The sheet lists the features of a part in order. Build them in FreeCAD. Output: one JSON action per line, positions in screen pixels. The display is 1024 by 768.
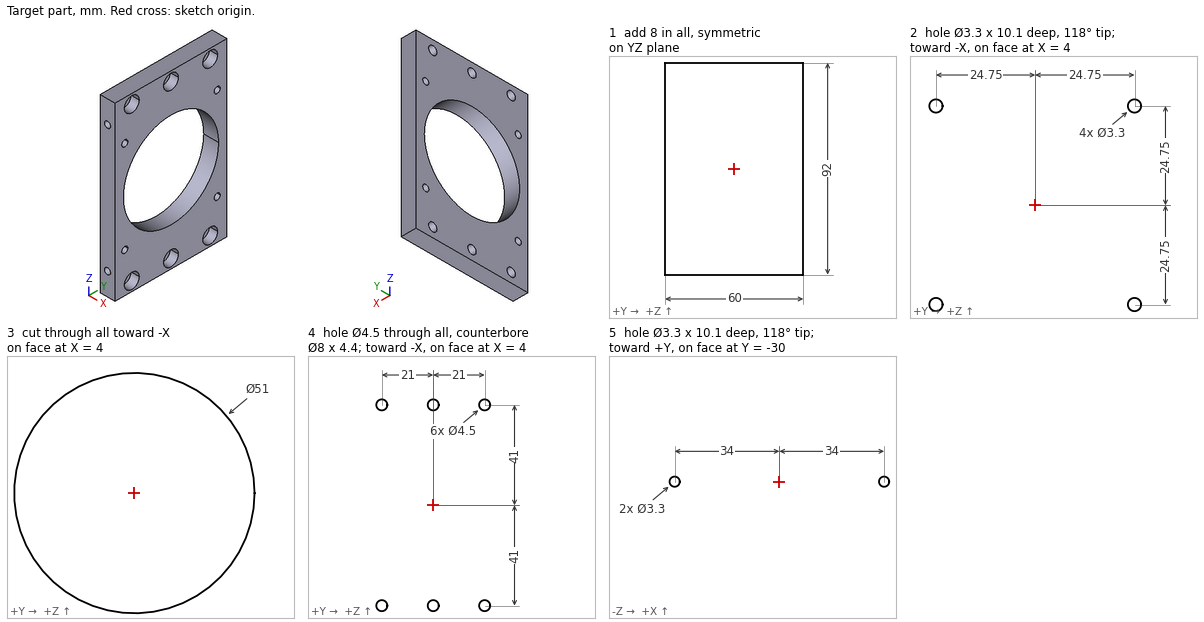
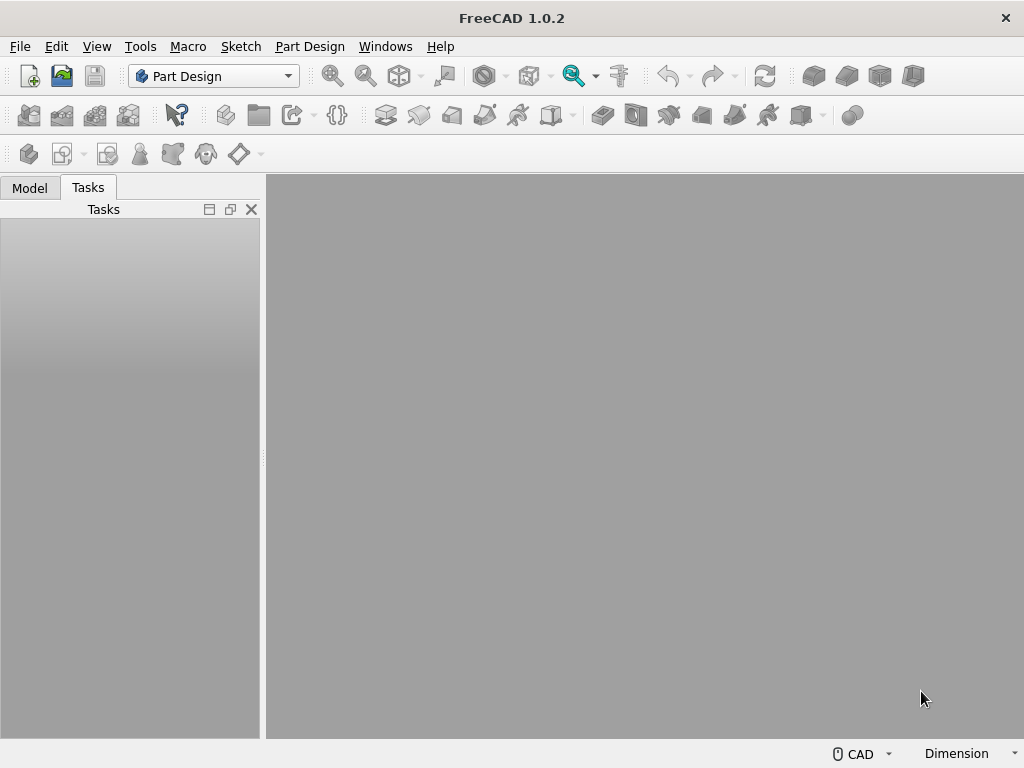
{"action": "left_click", "coordinate": [29, 76]}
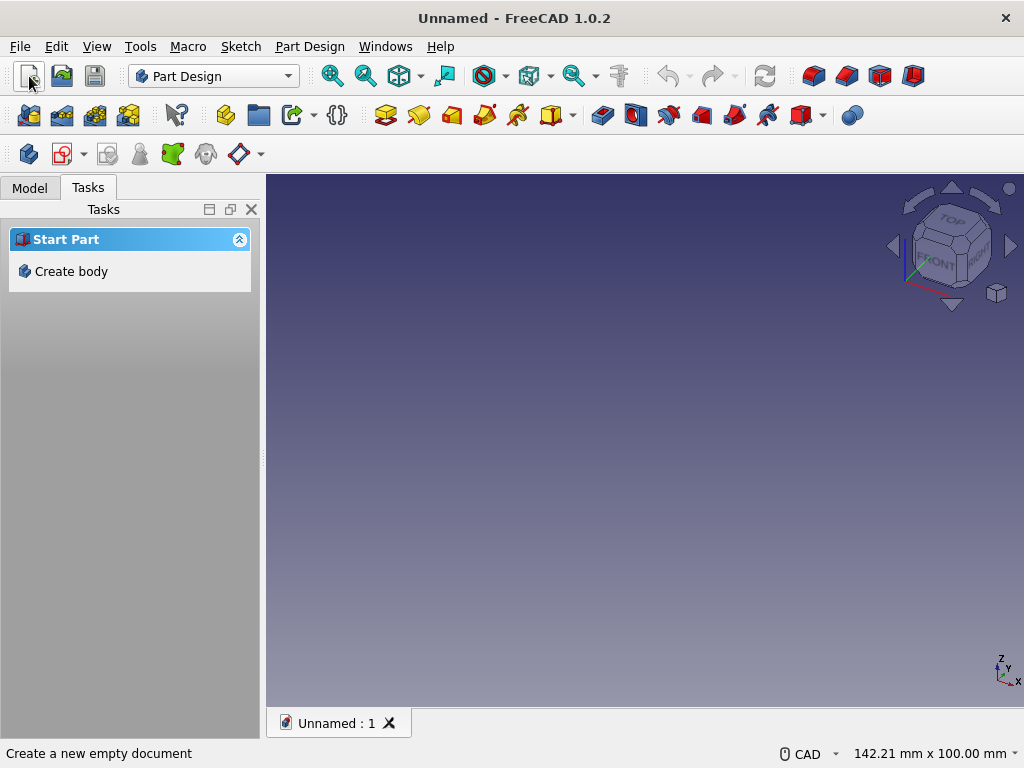
{"action": "left_click", "coordinate": [62, 154]}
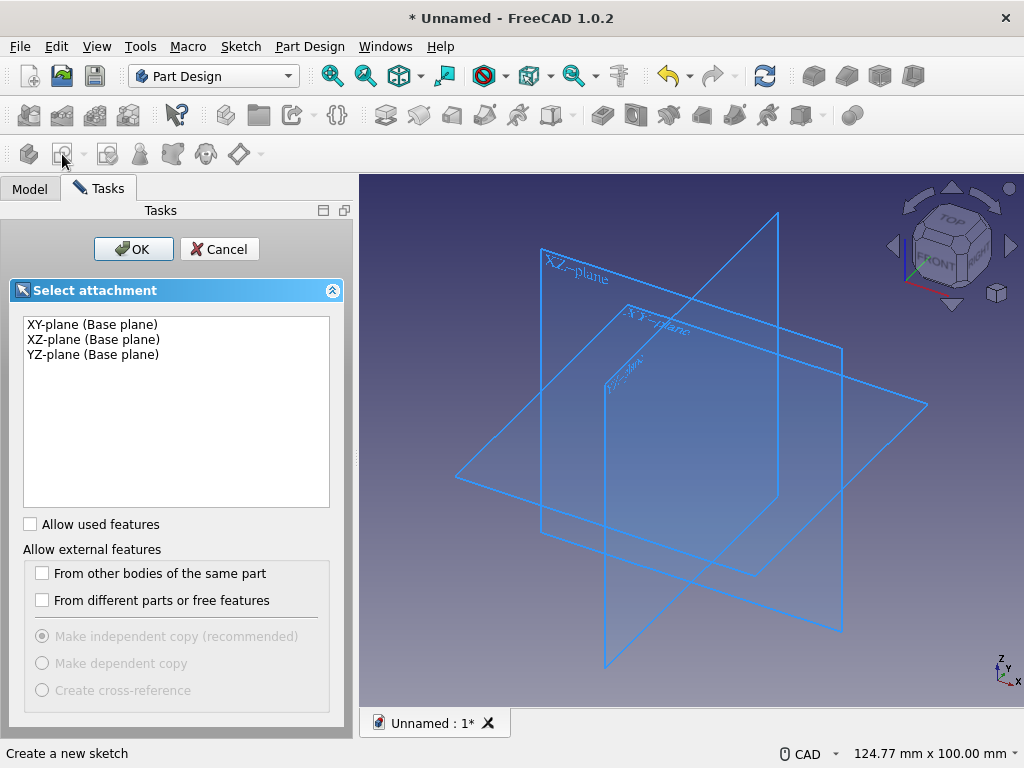
{"action": "left_click", "coordinate": [84, 354]}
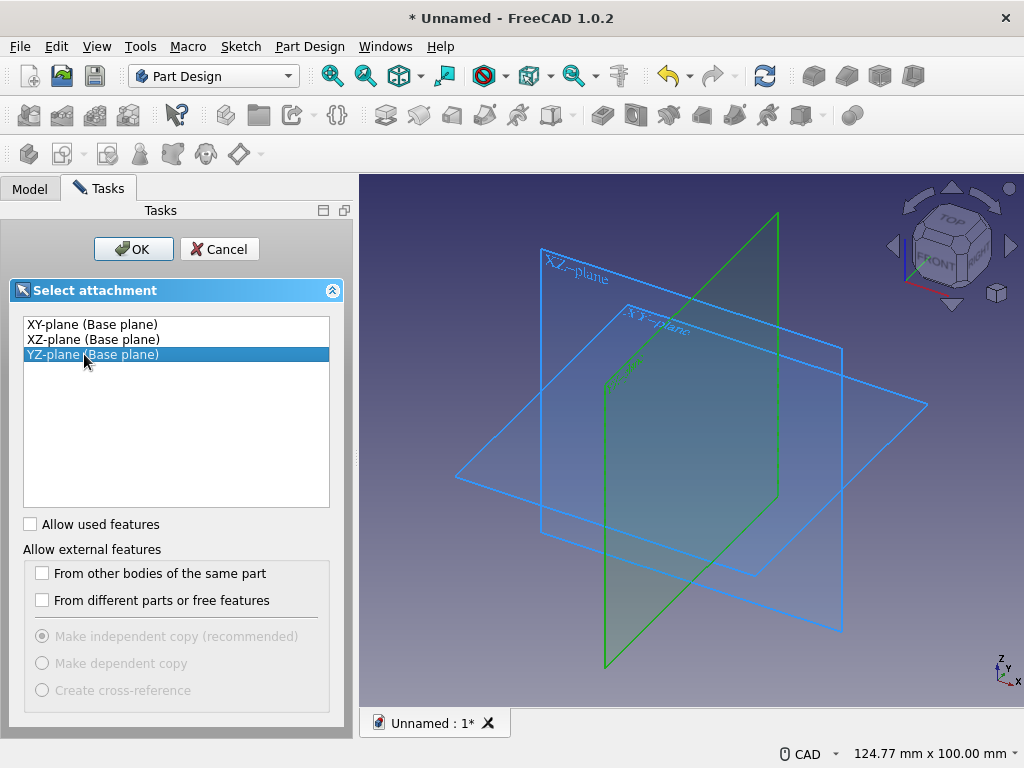
{"action": "left_click", "coordinate": [134, 249]}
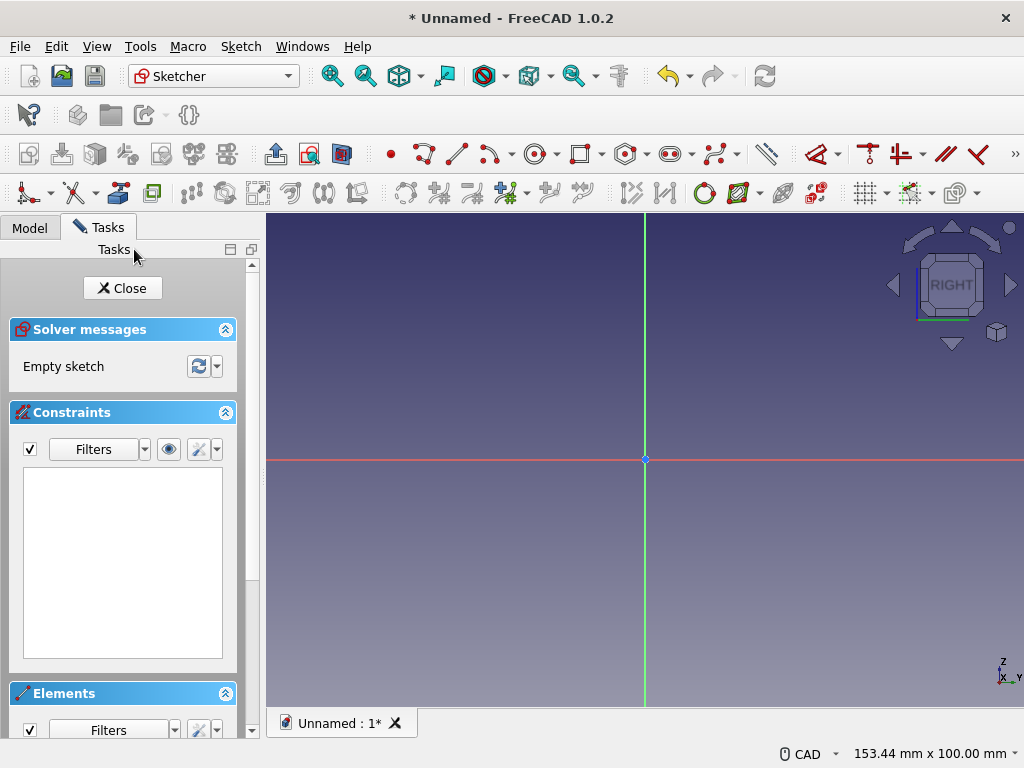
{"action": "scroll", "coordinate": [437, 460], "scroll_direction": "down", "scroll_amount": 2}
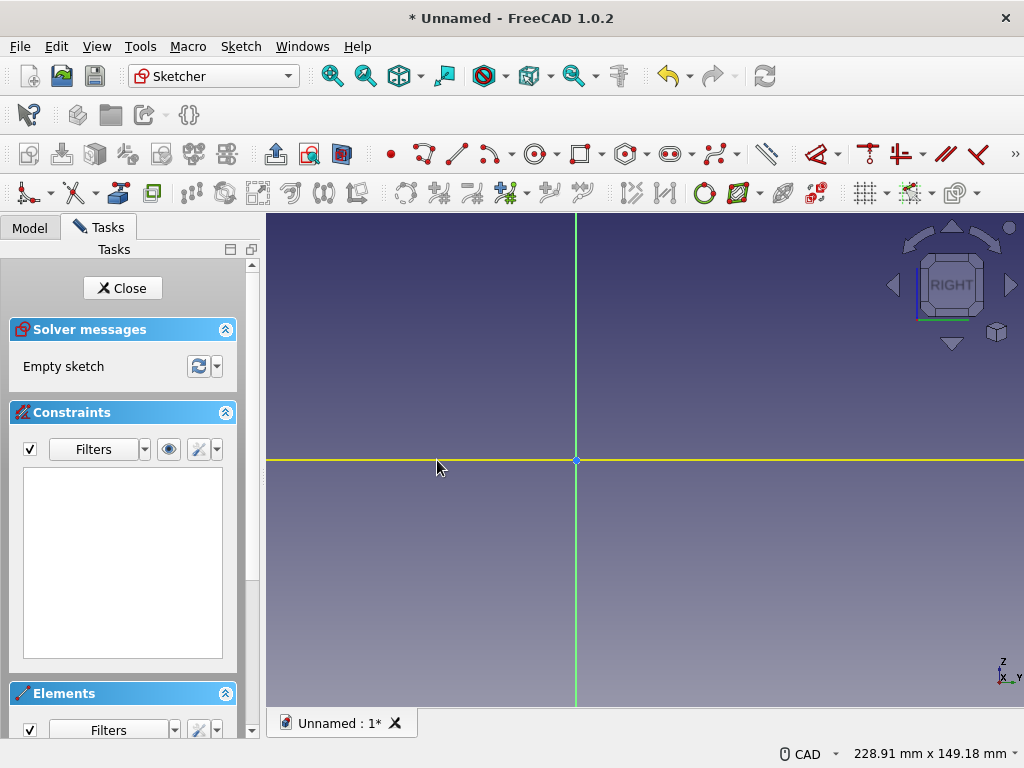
{"action": "key", "text": "g v"}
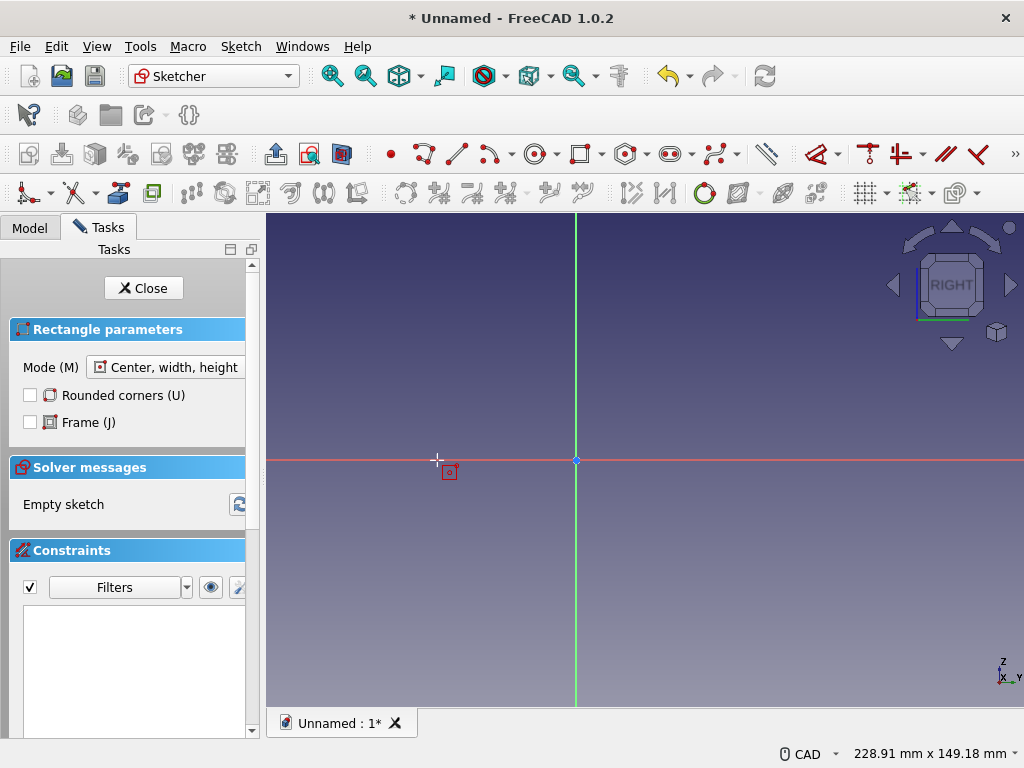
{"action": "left_click", "coordinate": [577, 460]}
{"action": "left_click", "coordinate": [676, 308]}
{"action": "key", "text": "Escape"}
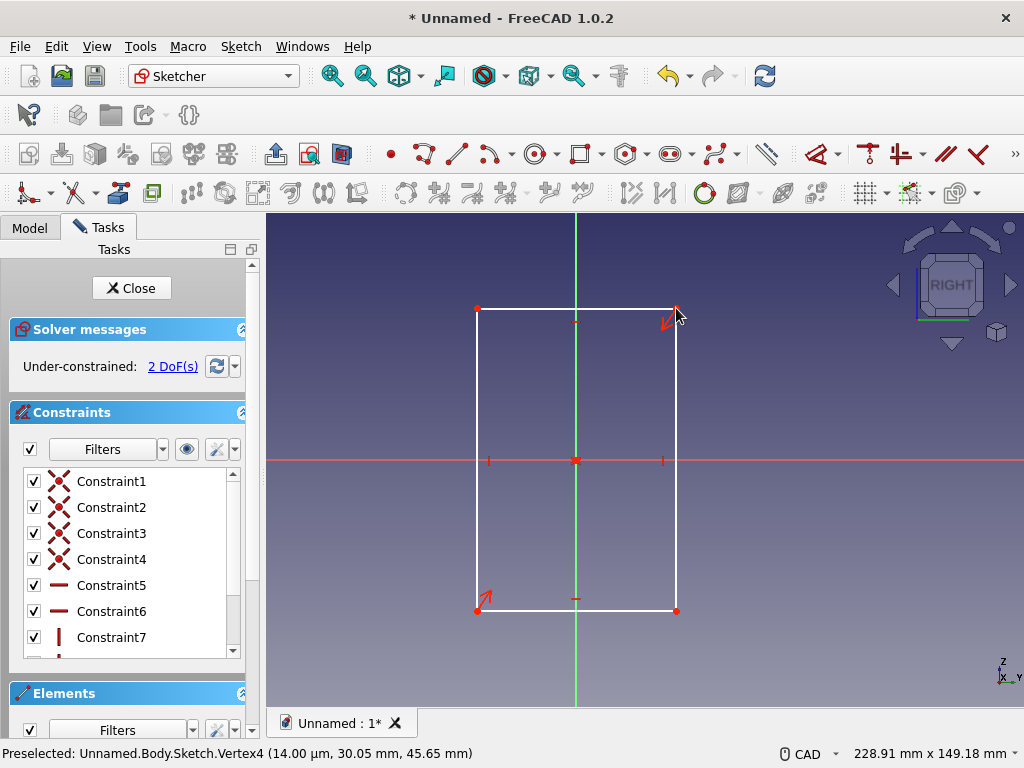
{"action": "left_click", "coordinate": [816, 154]}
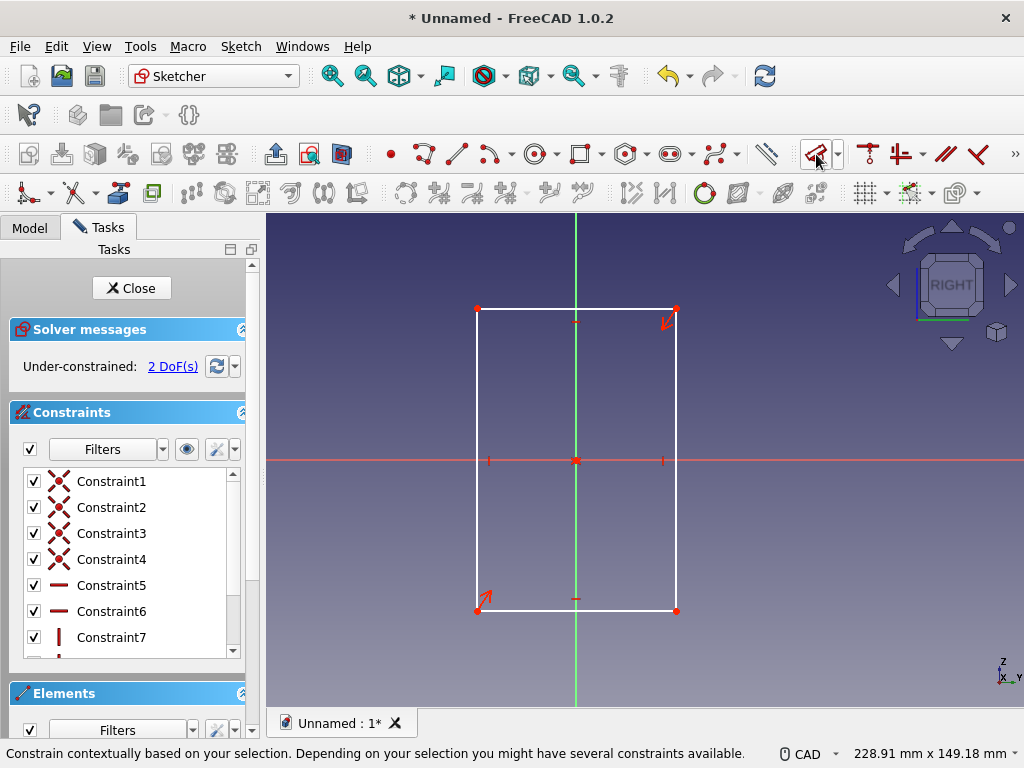
{"action": "left_click", "coordinate": [537, 611]}
{"action": "left_click", "coordinate": [531, 645]}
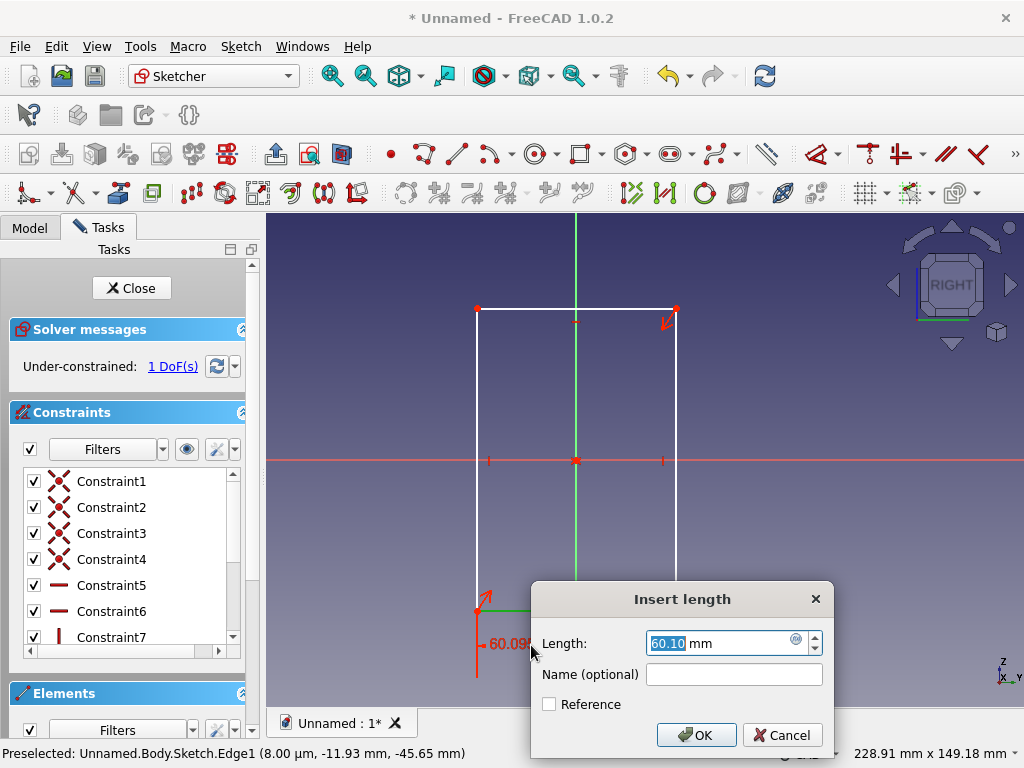
{"action": "type", "text": "60"}
{"action": "key", "text": "Return"}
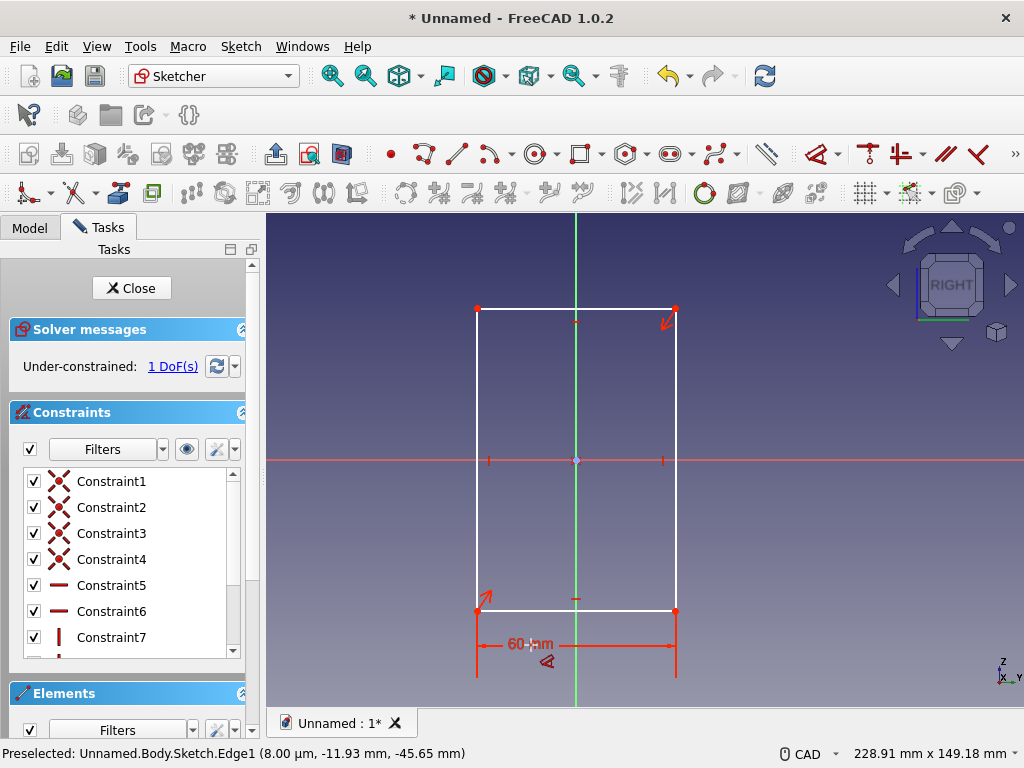
{"action": "left_click", "coordinate": [676, 521]}
{"action": "left_click", "coordinate": [710, 391]}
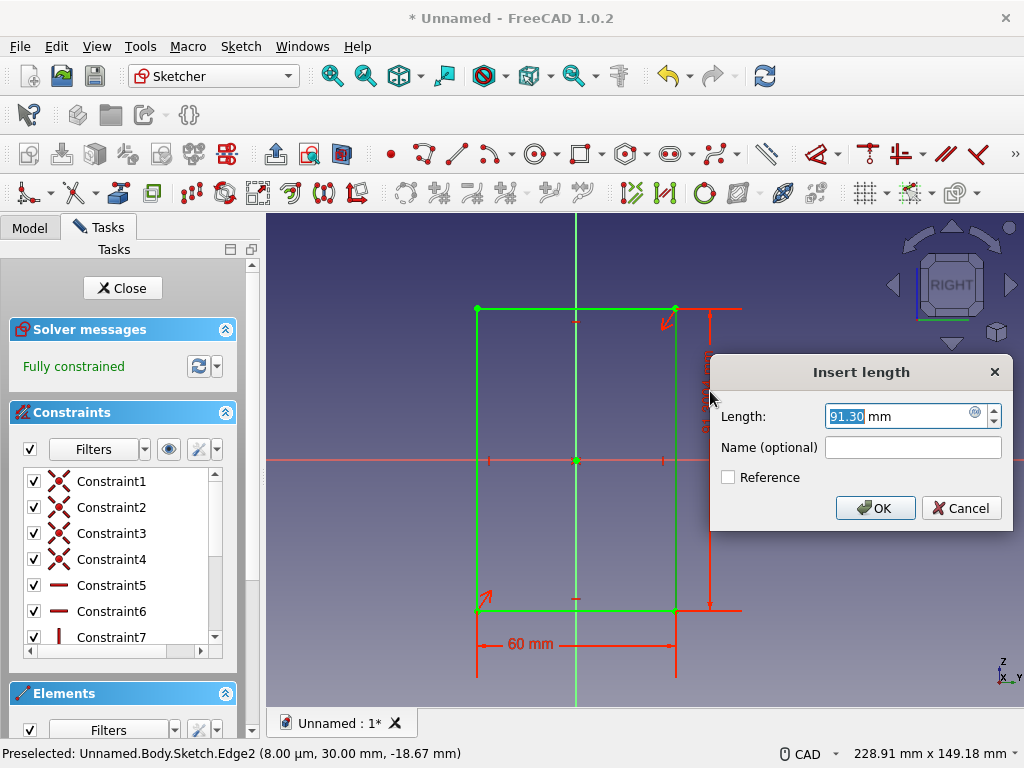
{"action": "type", "text": "92"}
{"action": "key", "text": "Return"}
{"action": "key", "text": "Escape"}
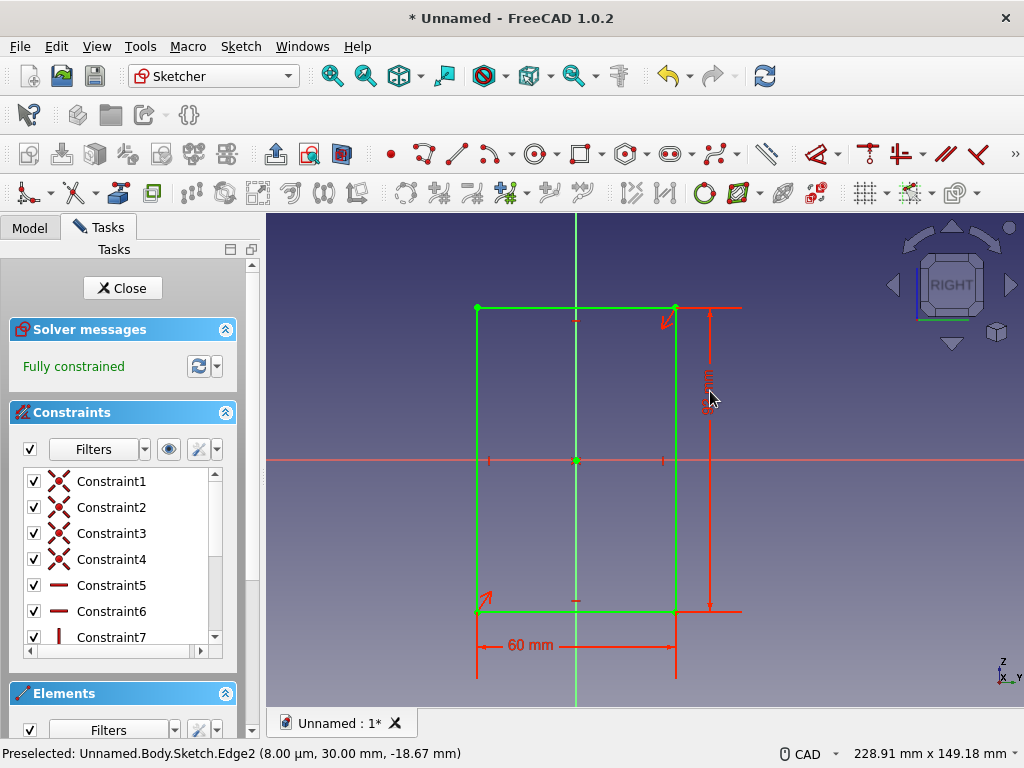
{"action": "left_click", "coordinate": [123, 288]}